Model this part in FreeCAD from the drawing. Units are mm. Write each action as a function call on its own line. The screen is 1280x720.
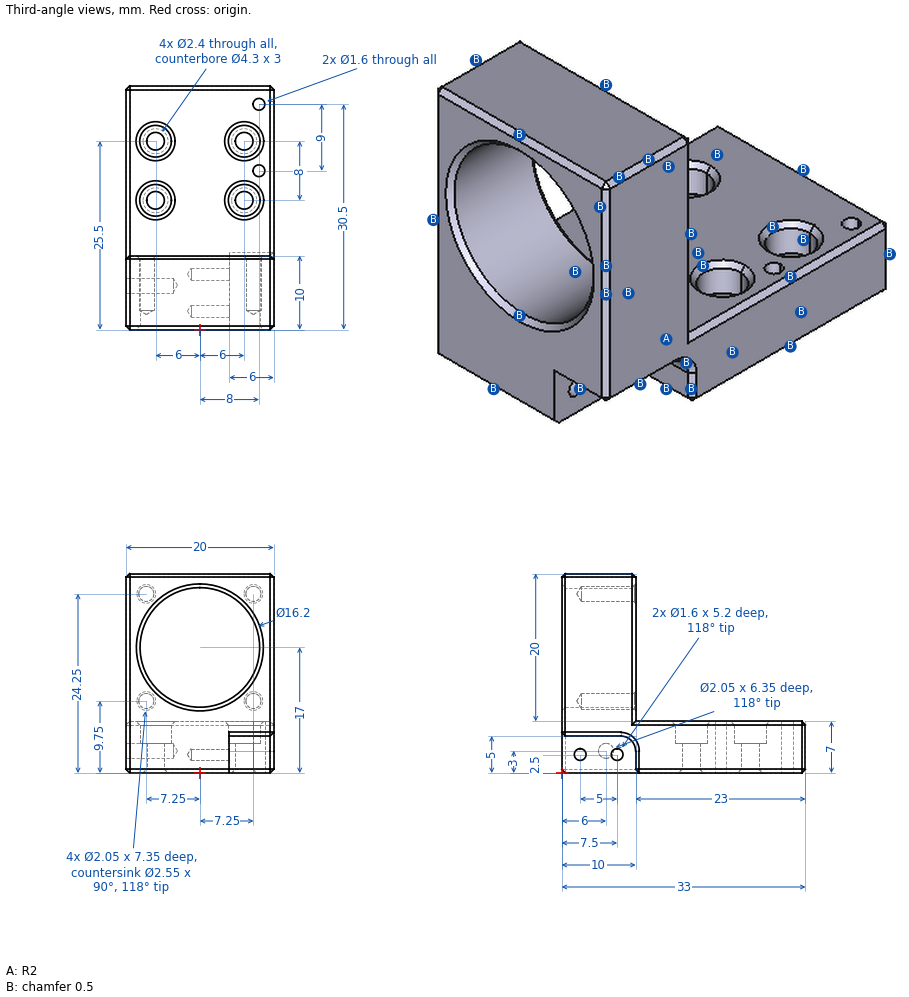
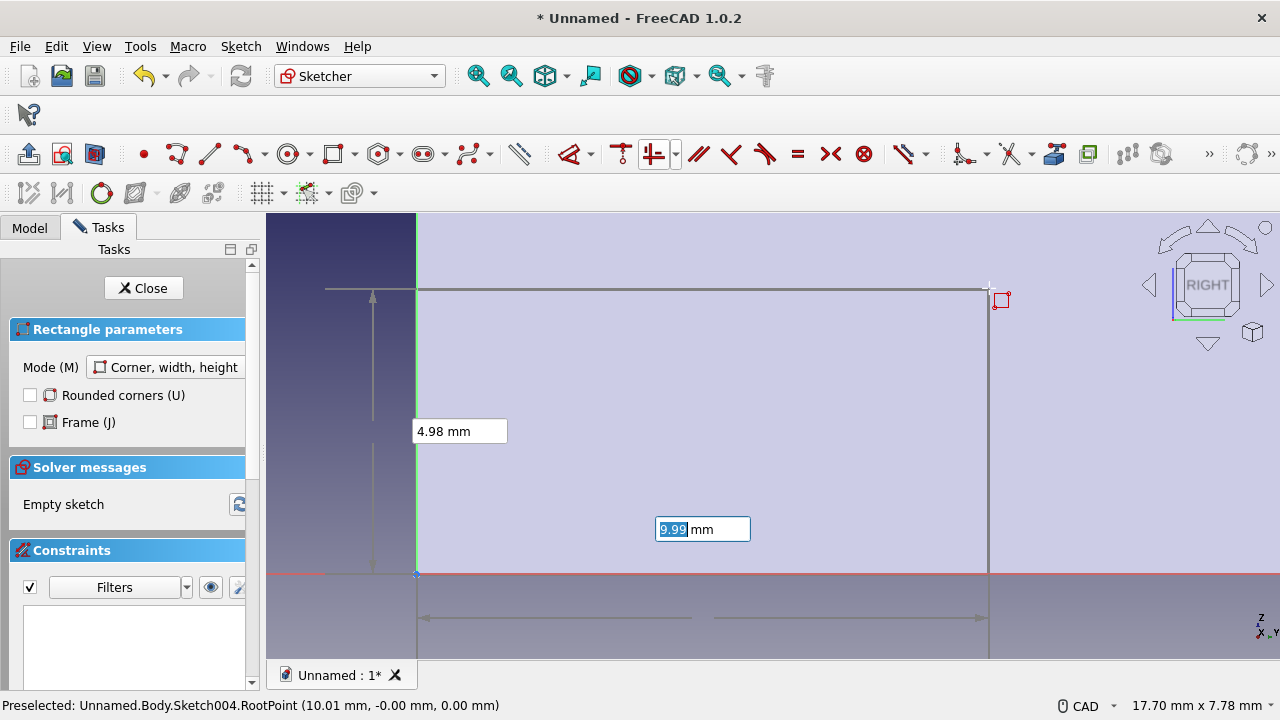
text(10)
key(Tab)
text(5)
key(Return)
key(Escape)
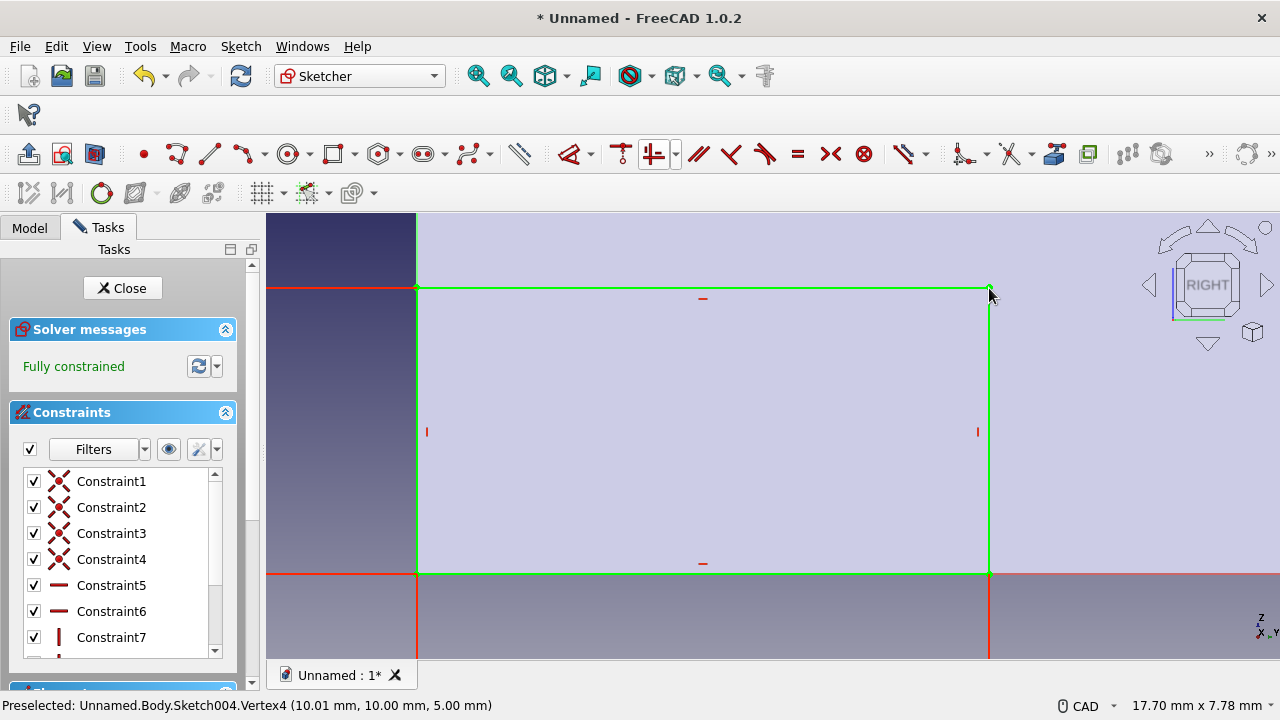
click(123, 288)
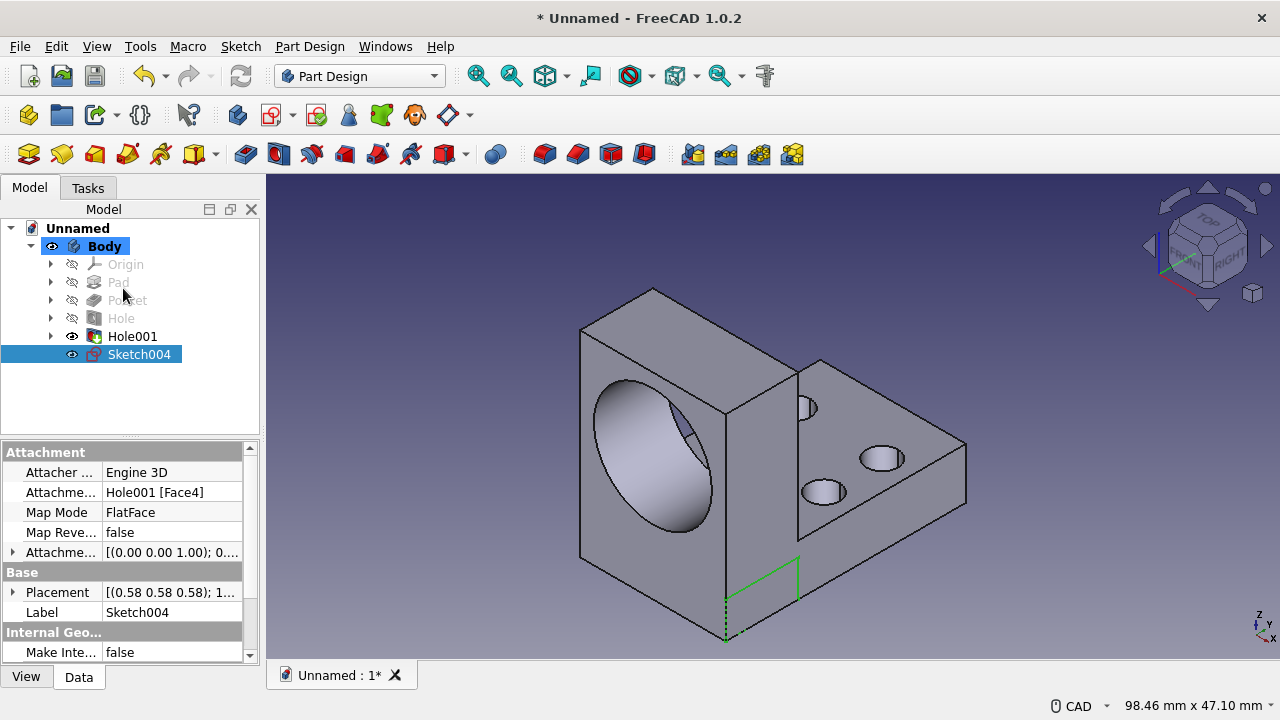
click(246, 154)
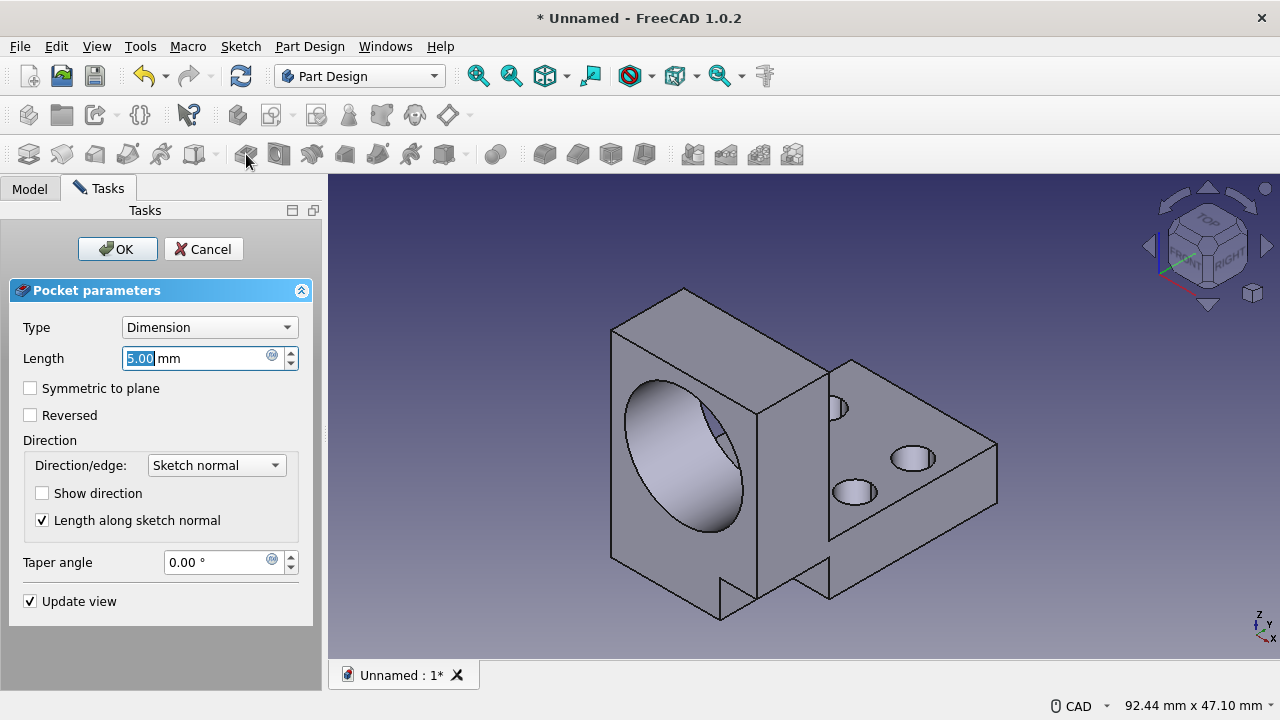
text(6)
key(Tab)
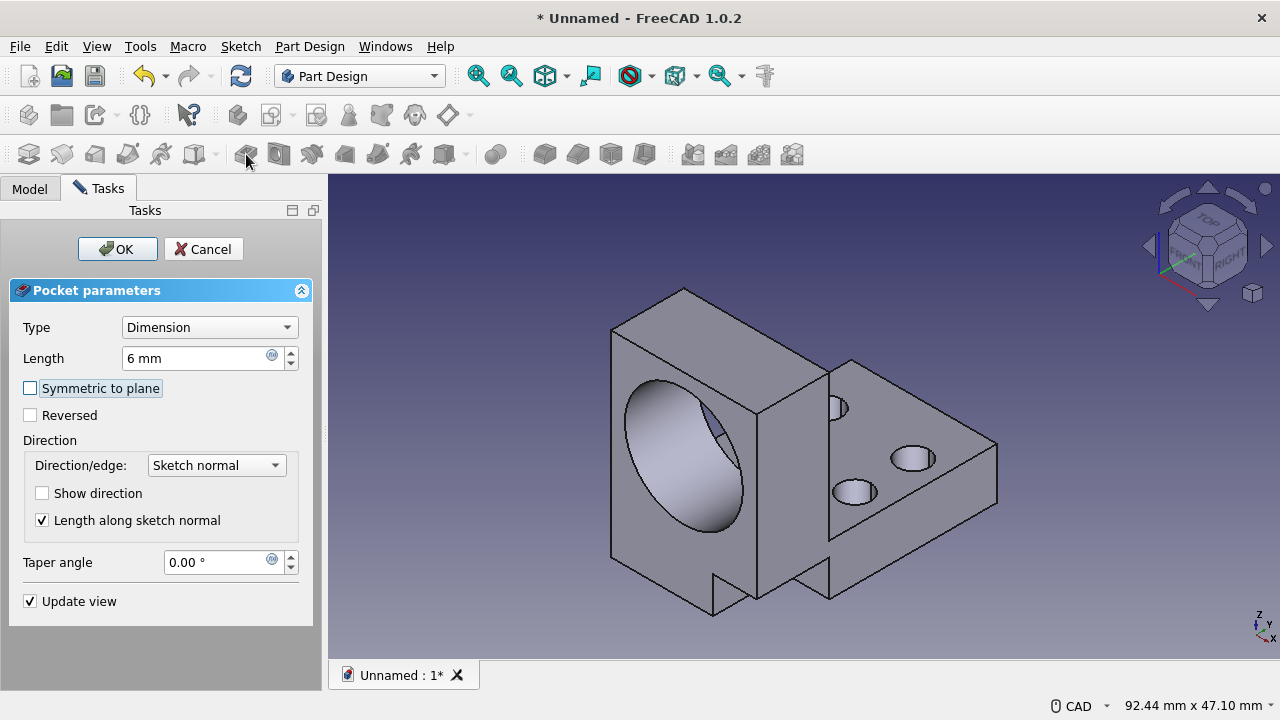
click(118, 249)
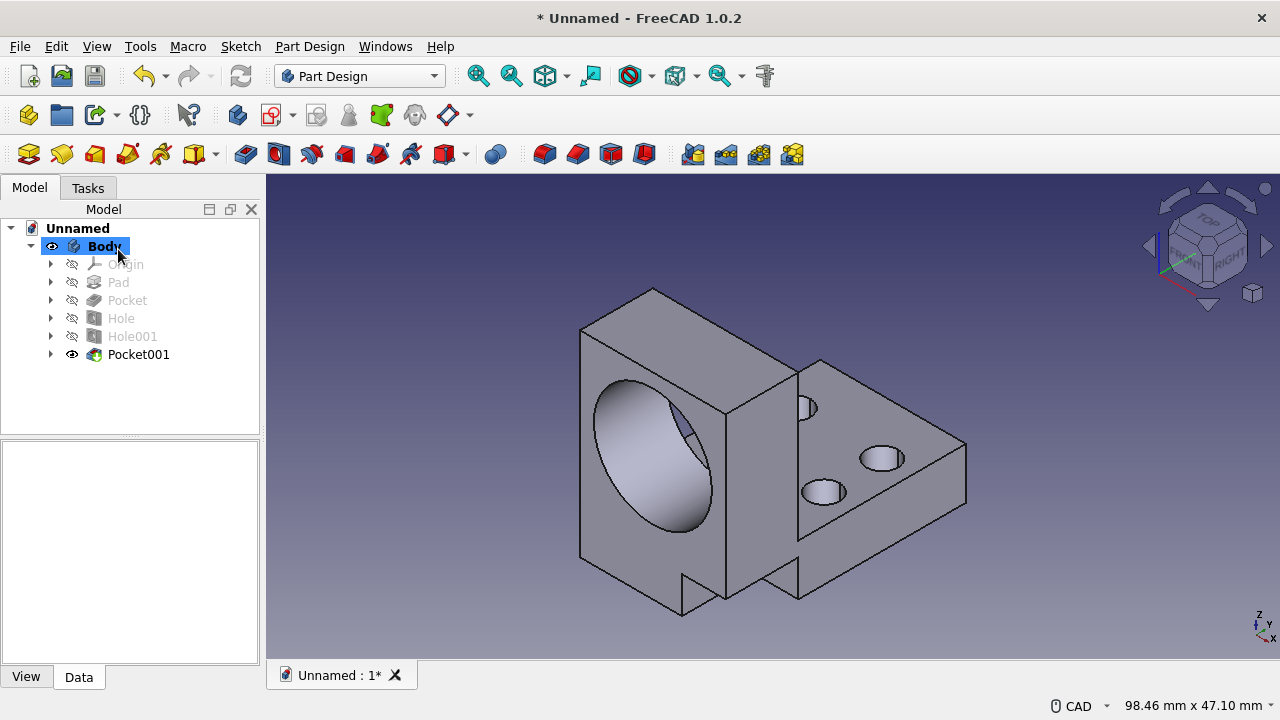
key(3)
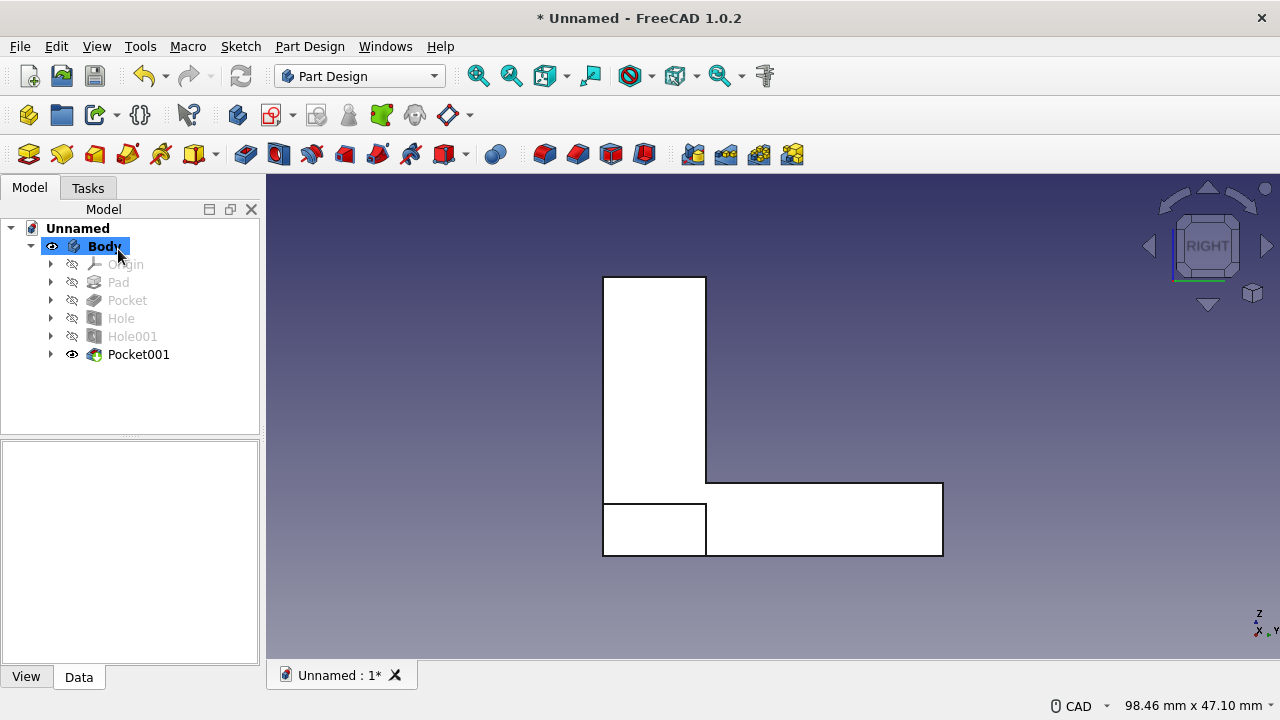
click(669, 529)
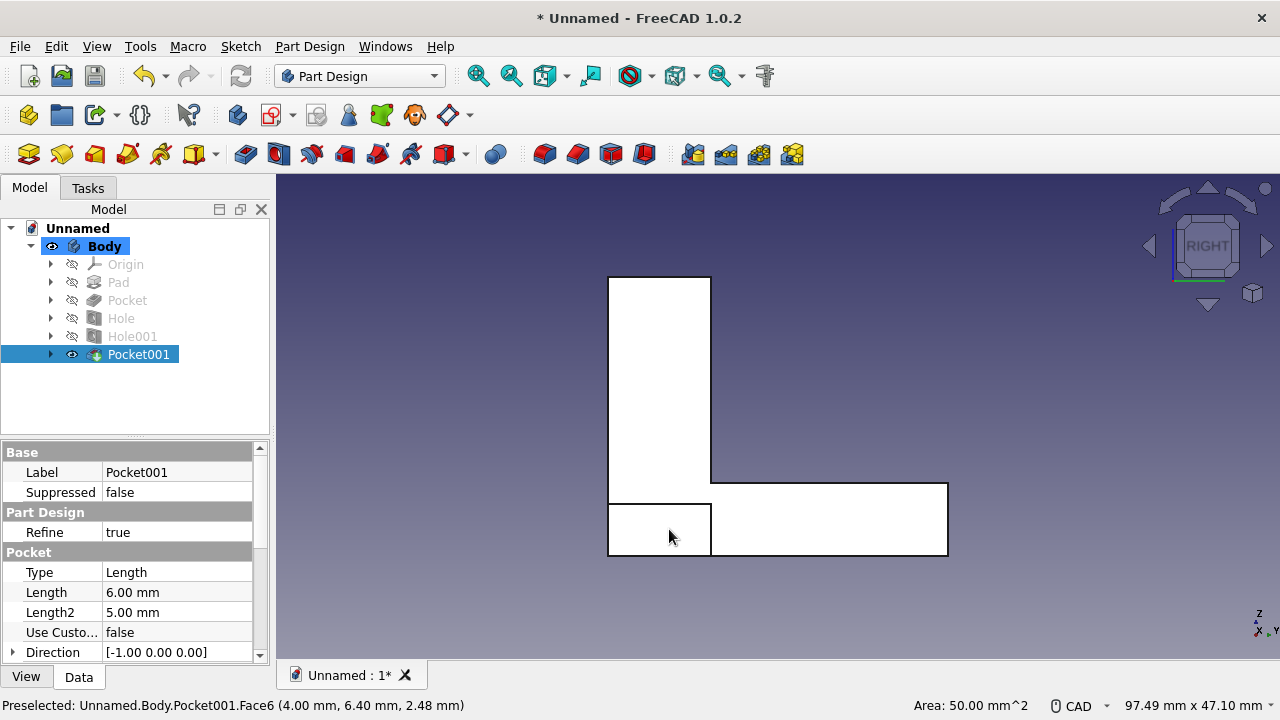
click(270, 116)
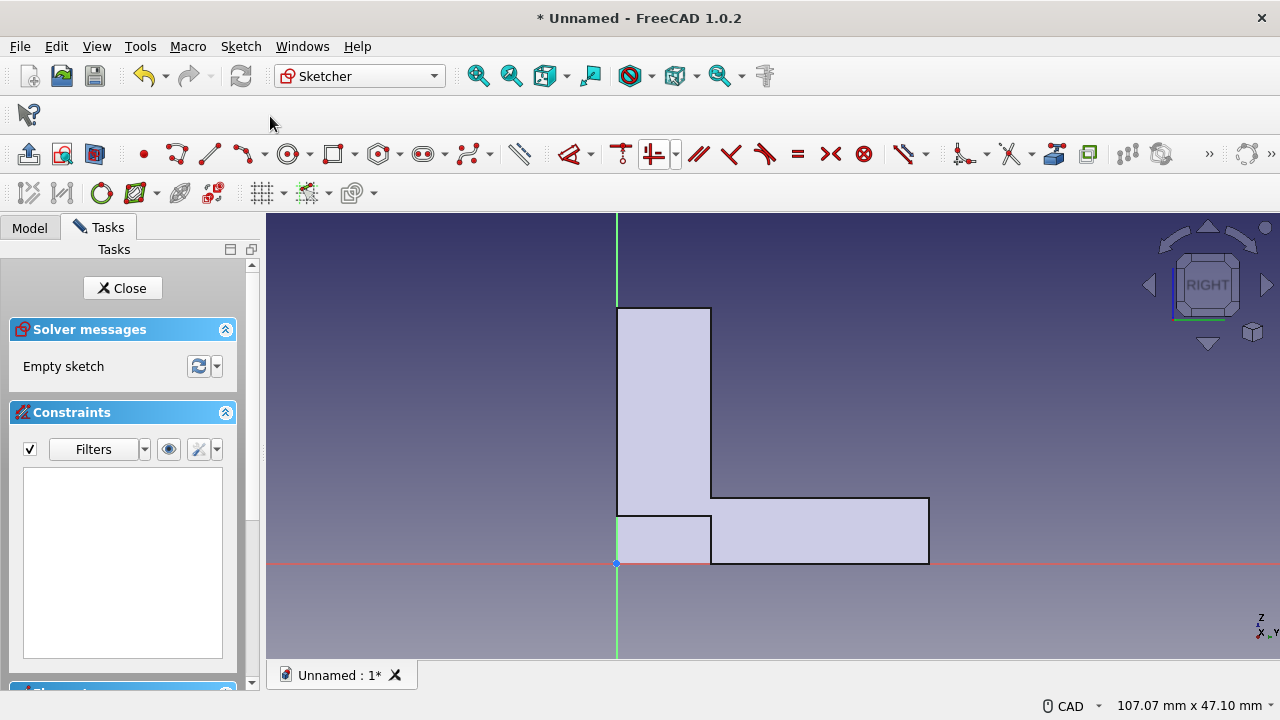
key(q)
key(s)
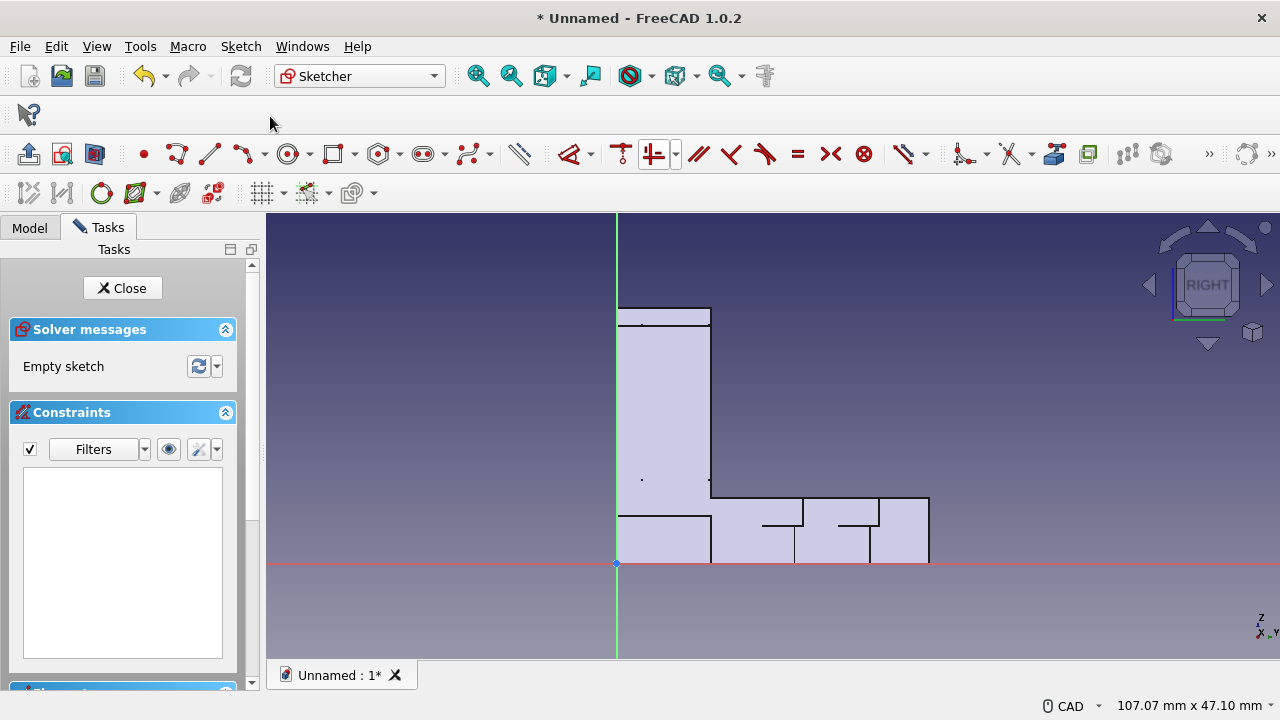
scroll(648, 566, up, 10)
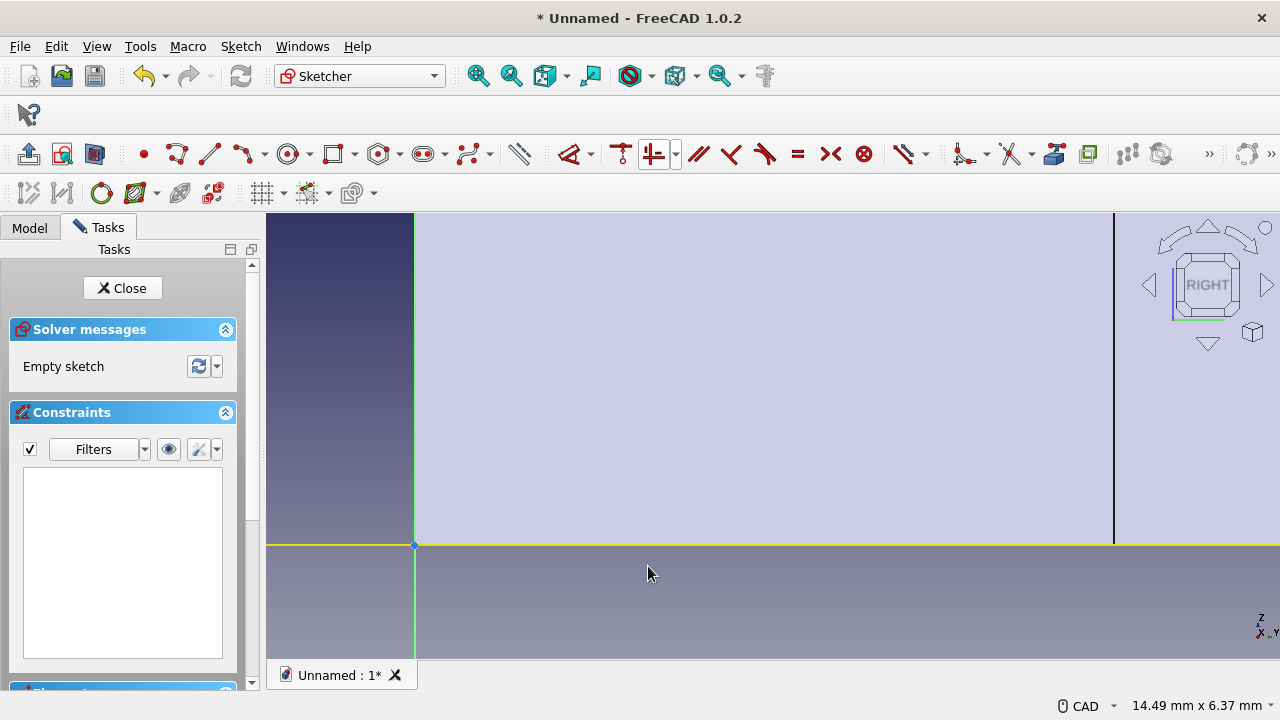
key(g)
key(c)